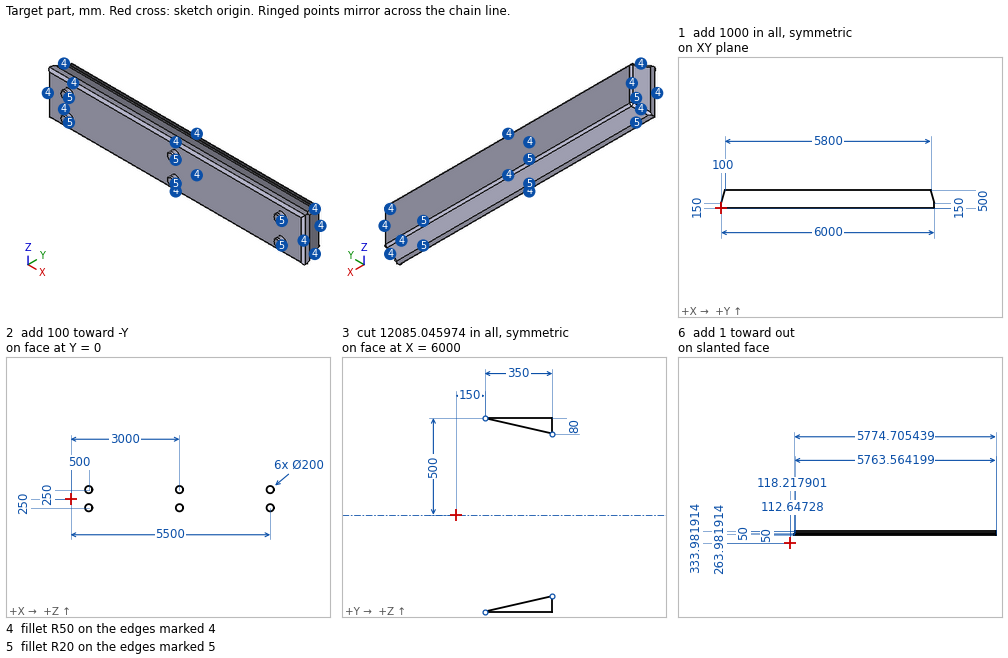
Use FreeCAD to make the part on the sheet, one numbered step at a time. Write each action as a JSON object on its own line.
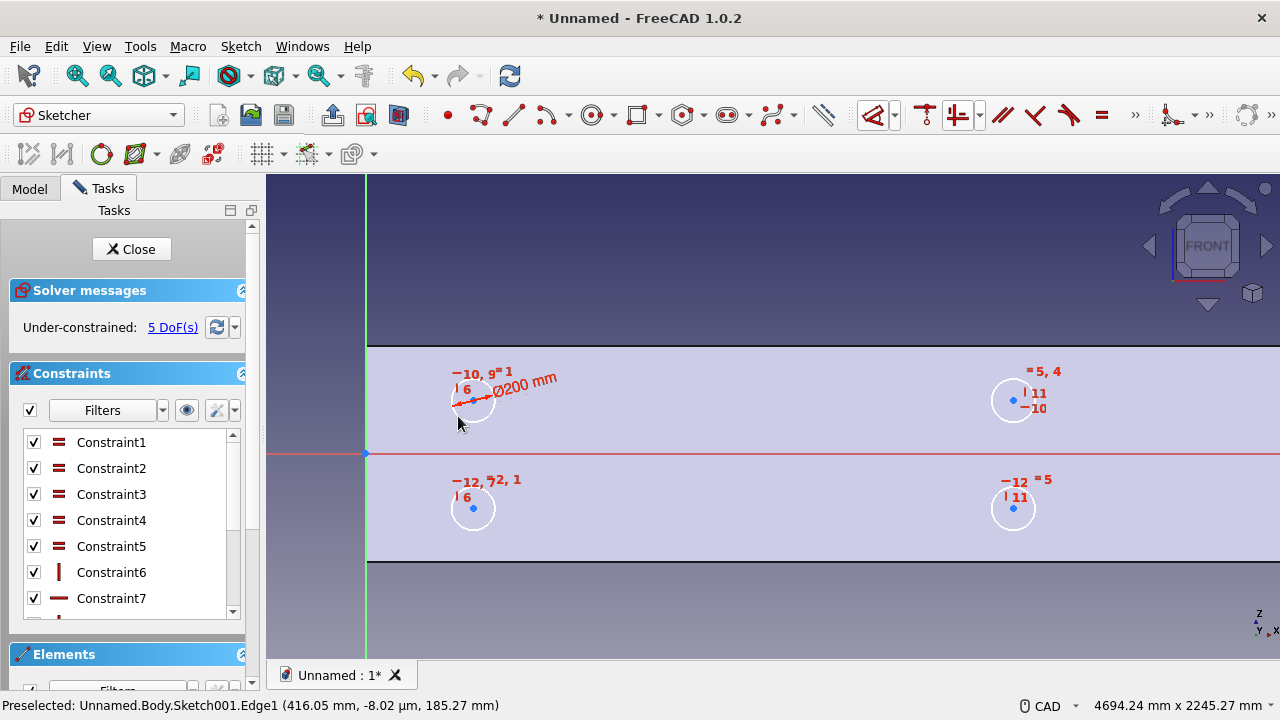
{"action": "left_click", "coordinate": [473, 401]}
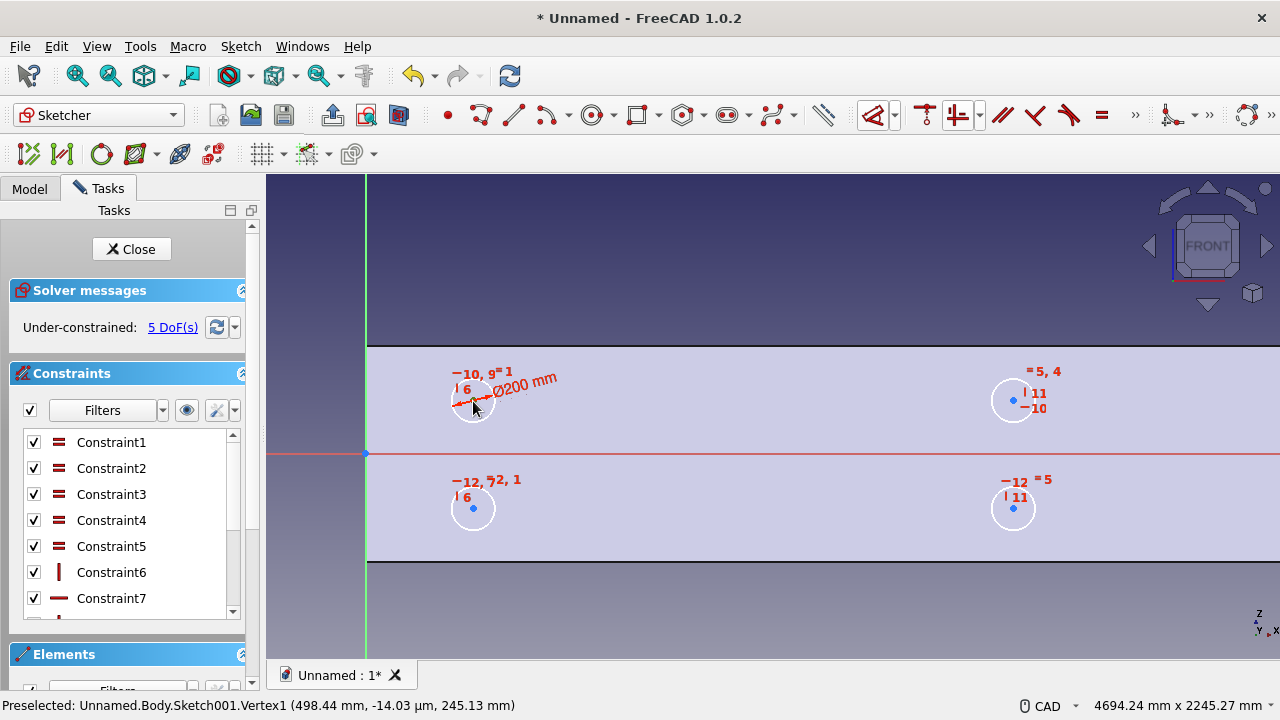
{"action": "key", "text": "l"}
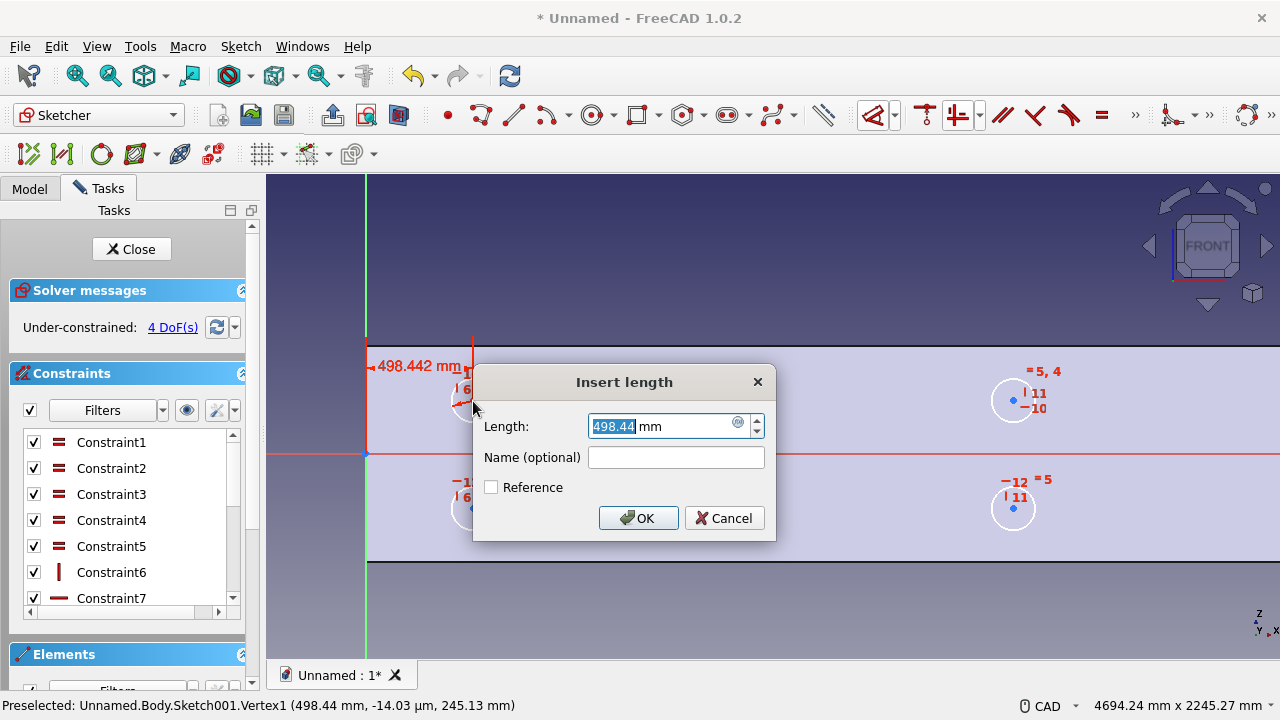
{"action": "type", "text": "500"}
{"action": "key", "text": "Return"}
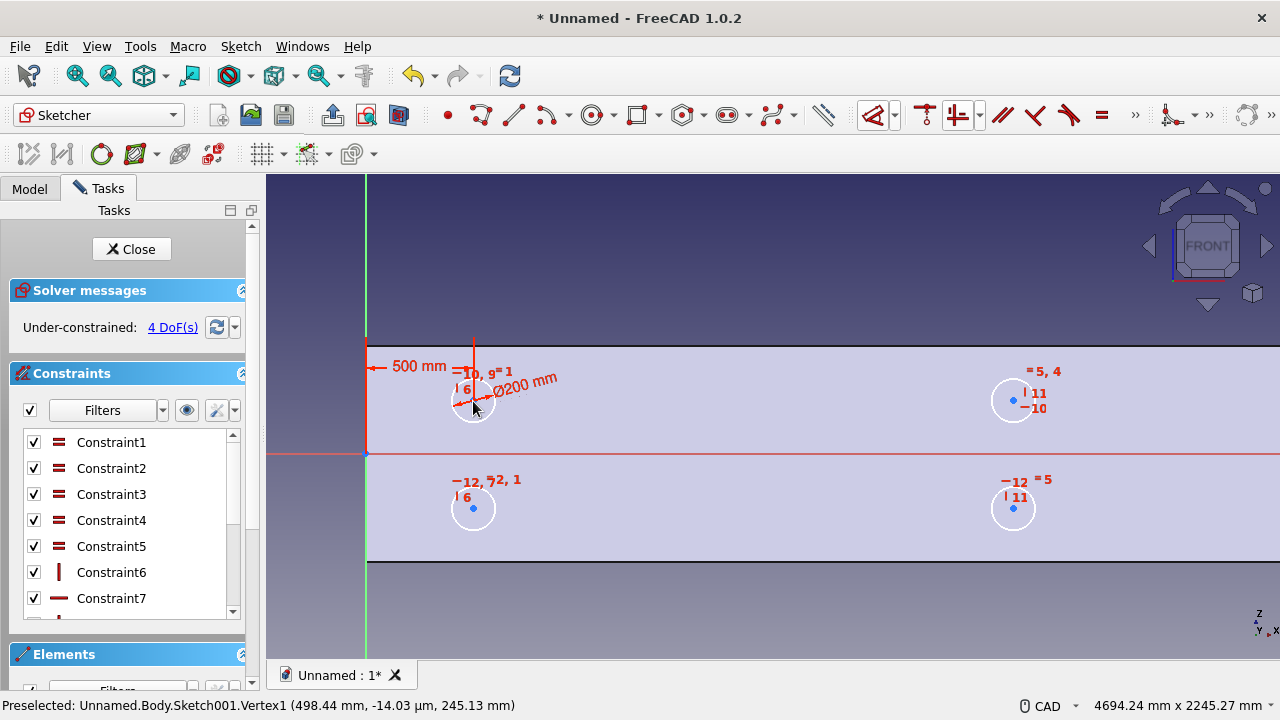
{"action": "left_click", "coordinate": [474, 401]}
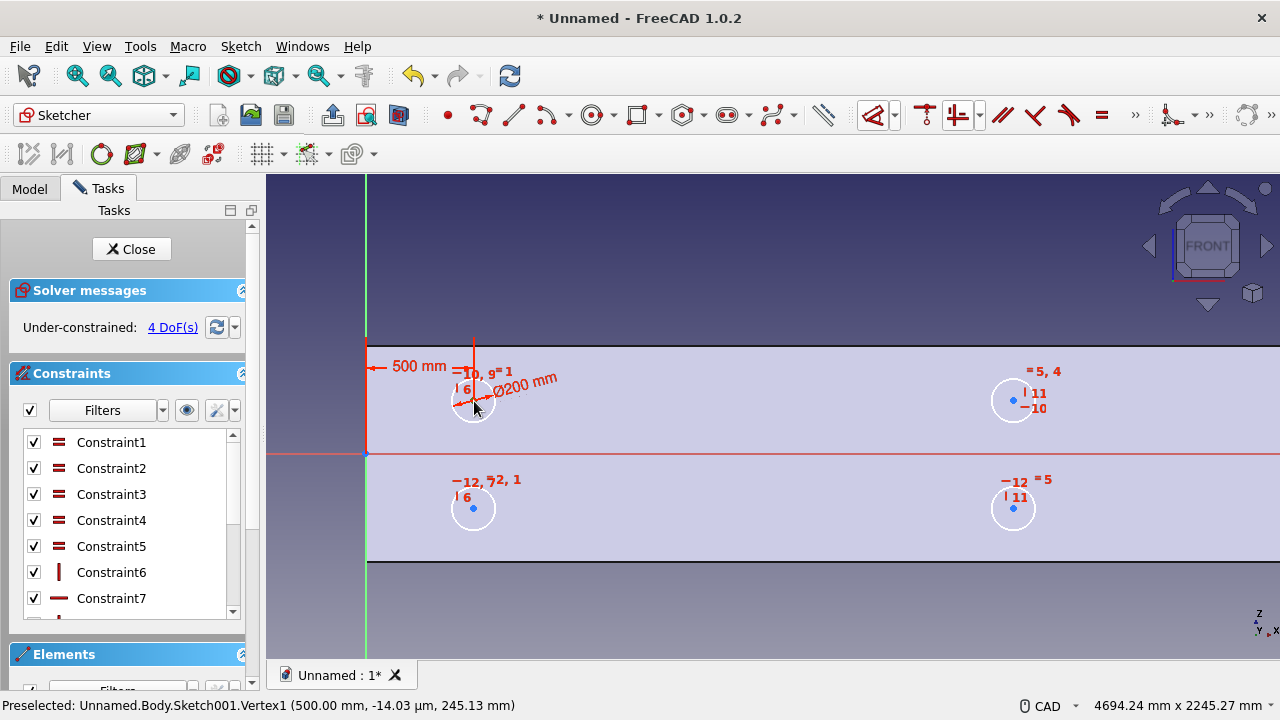
{"action": "left_click", "coordinate": [894, 116]}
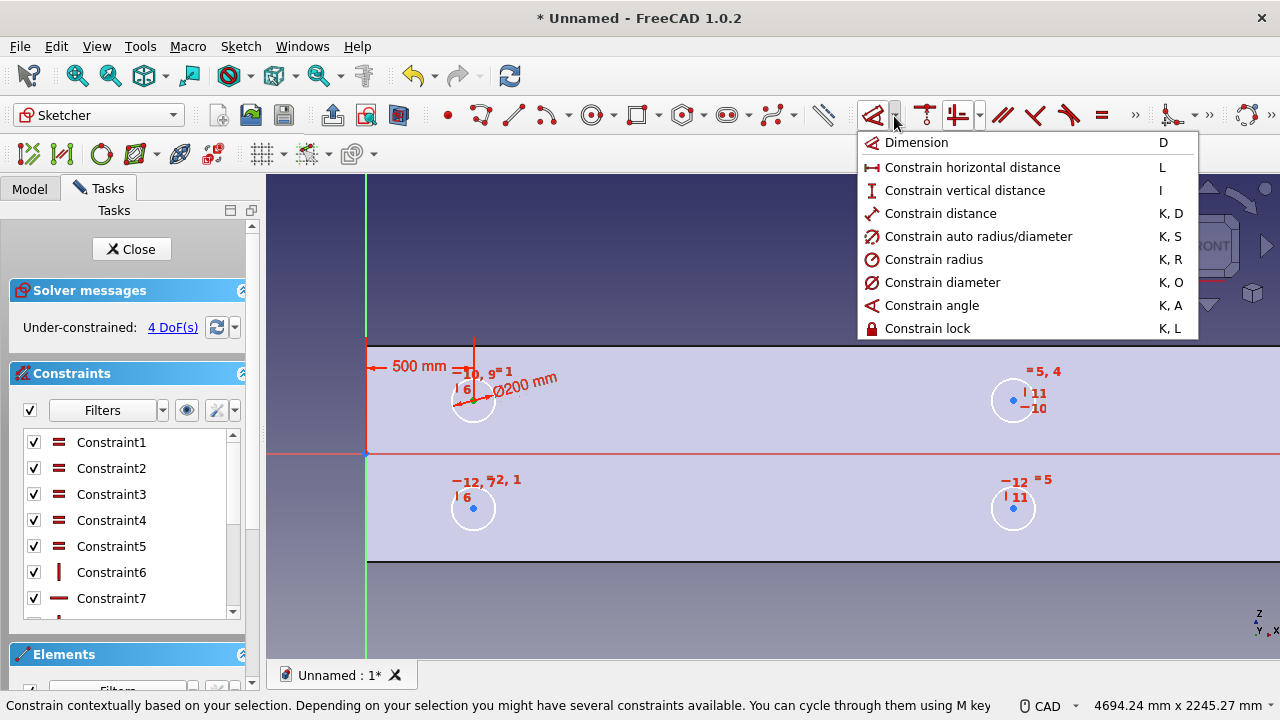
{"action": "left_click", "coordinate": [1028, 190]}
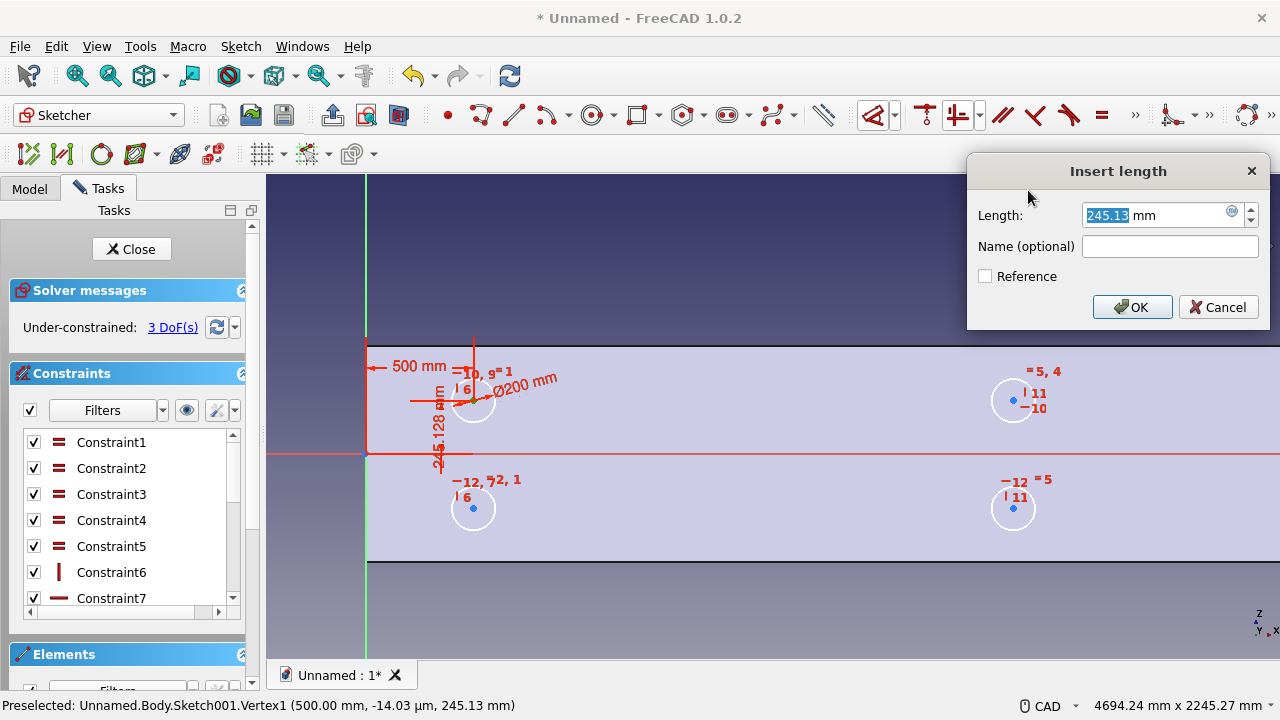
{"action": "type", "text": "250"}
{"action": "key", "text": "Return"}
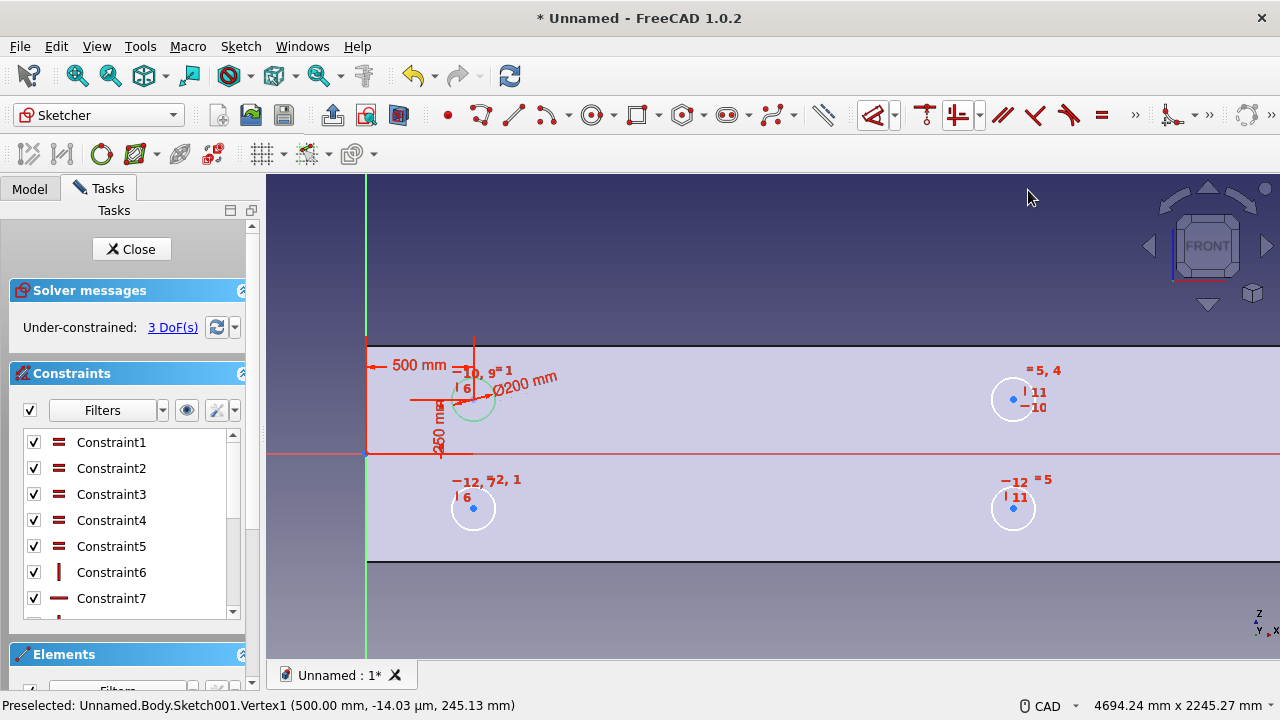
{"action": "left_click", "coordinate": [474, 509]}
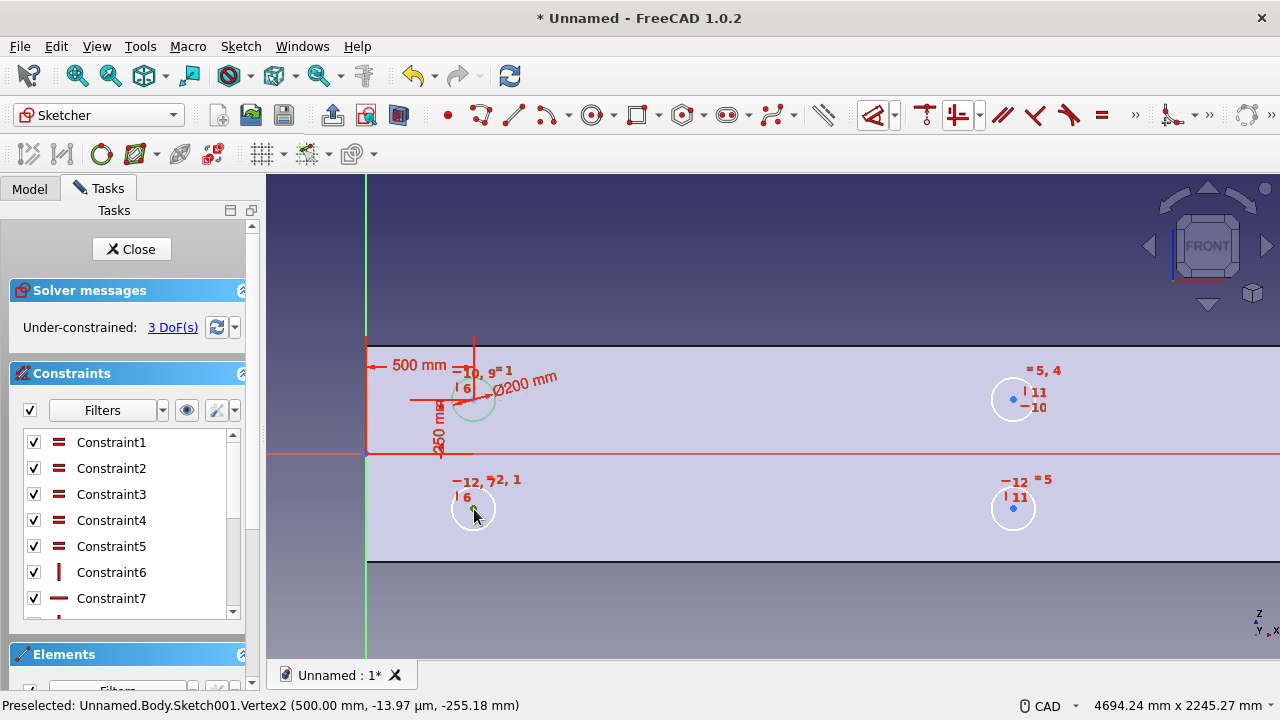
{"action": "key", "text": "i"}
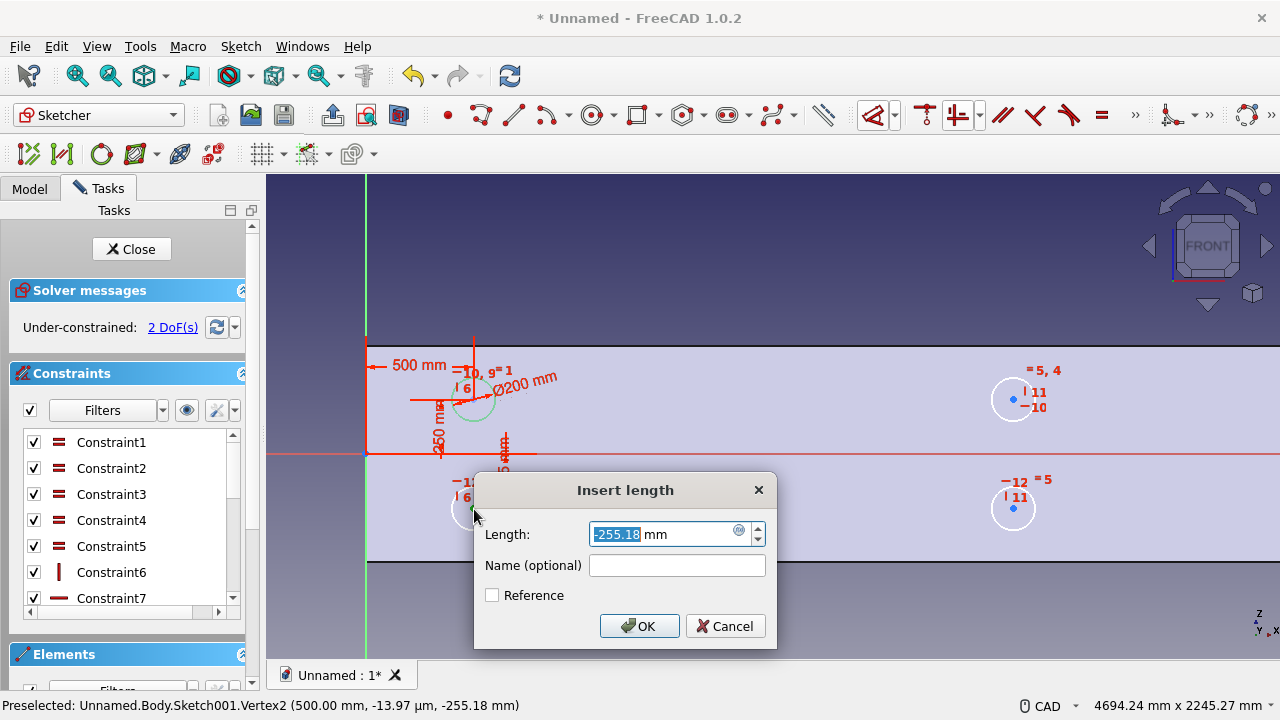
{"action": "type", "text": "-250"}
{"action": "key", "text": "Return"}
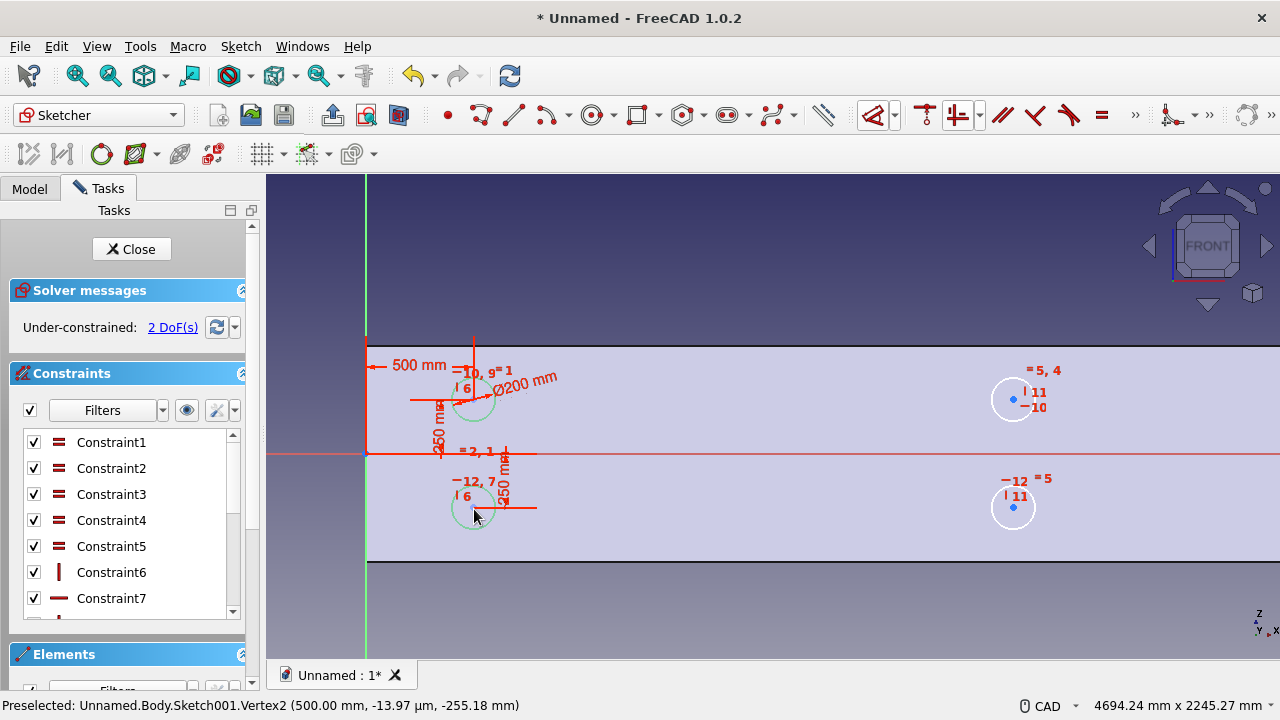
{"action": "scroll", "coordinate": [488, 386], "scroll_direction": "down", "scroll_amount": 4}